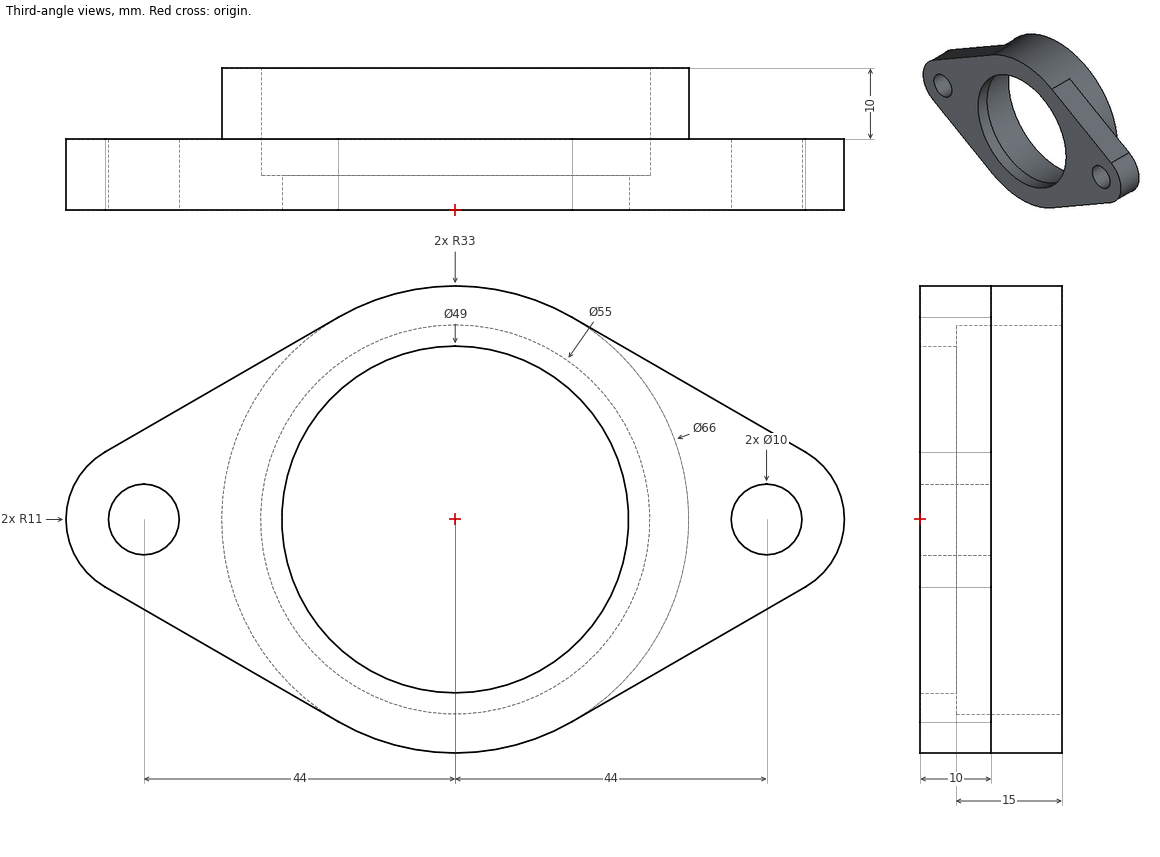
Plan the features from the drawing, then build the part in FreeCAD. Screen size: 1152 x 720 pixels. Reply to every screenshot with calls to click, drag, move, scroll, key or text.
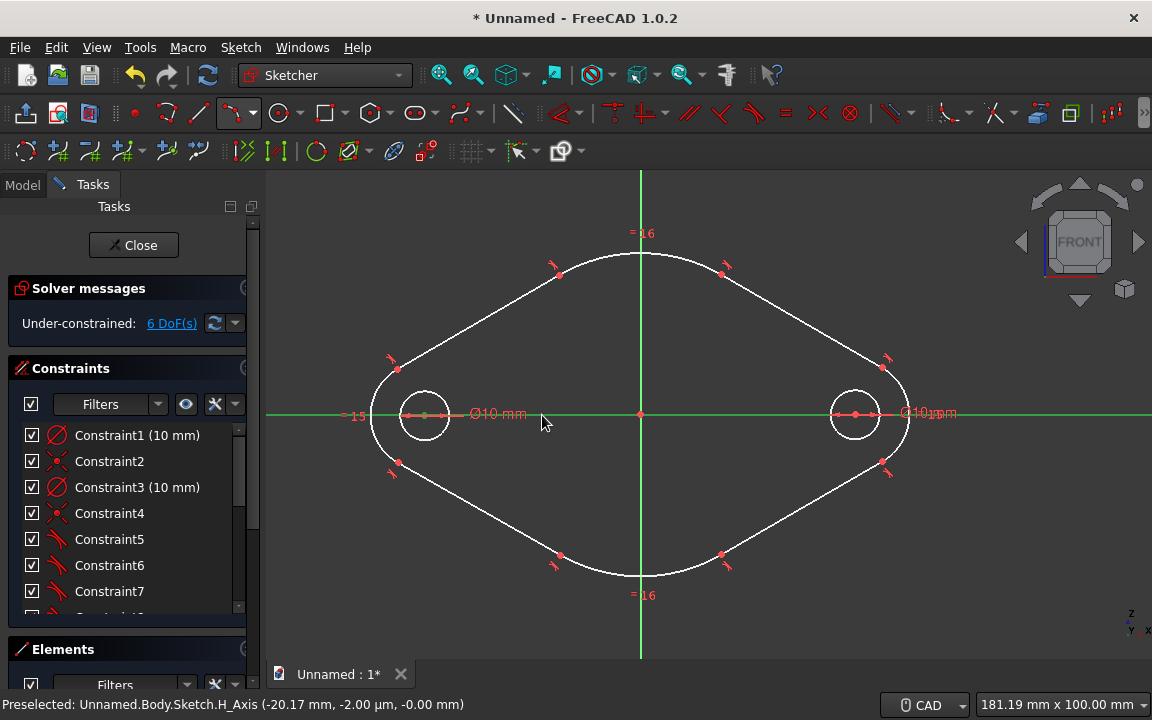
click(614, 114)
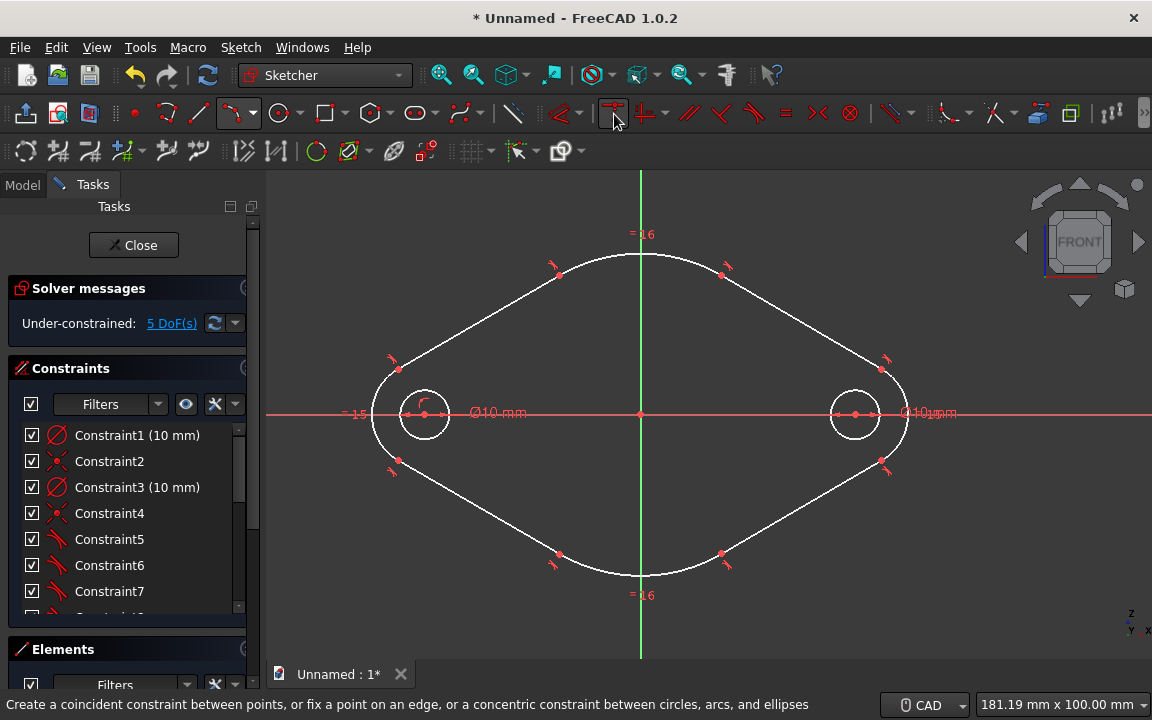
click(855, 415)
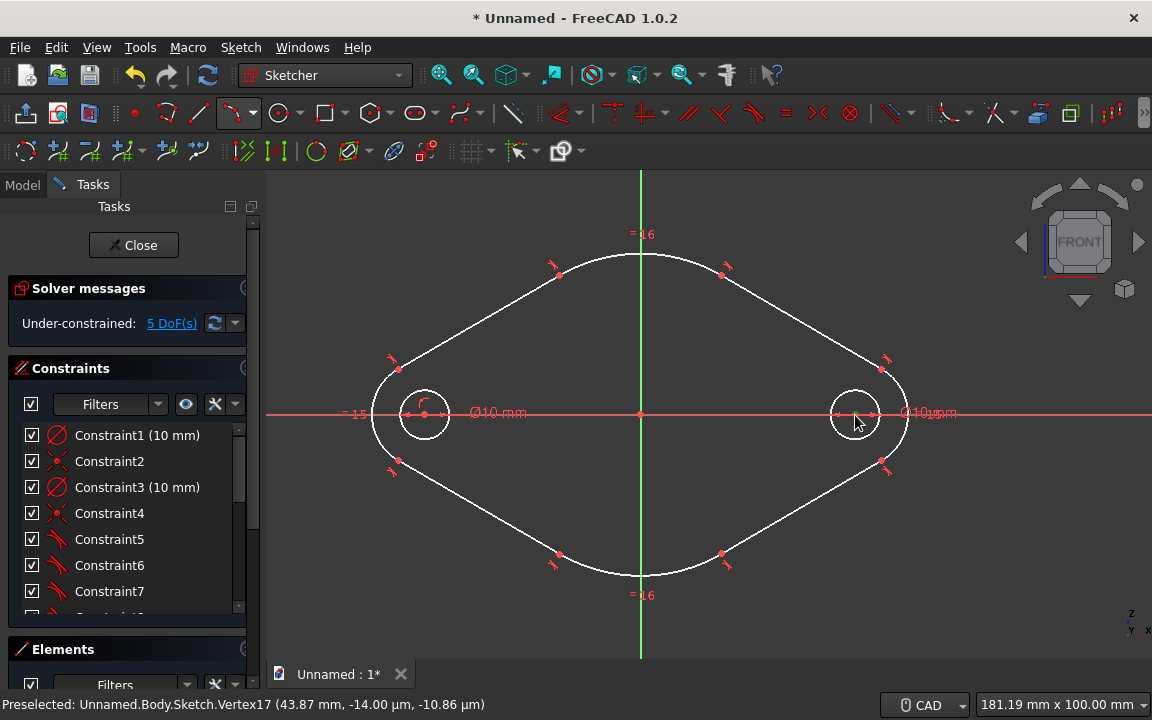
click(542, 415)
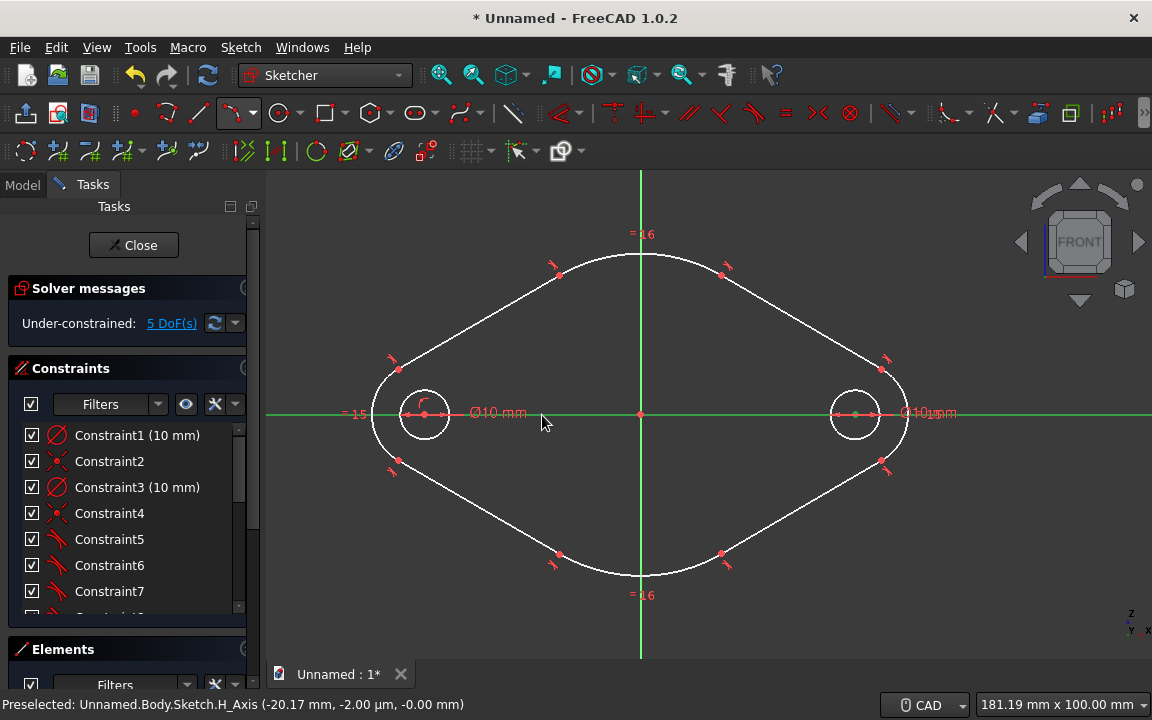
click(614, 114)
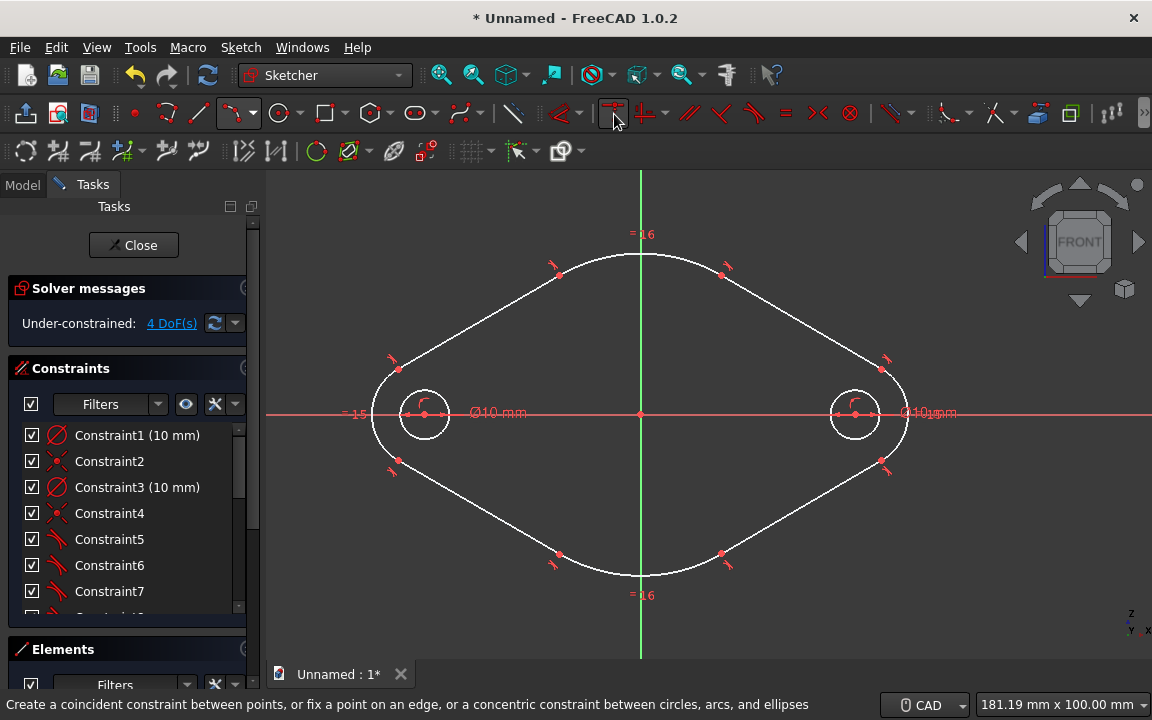
click(560, 114)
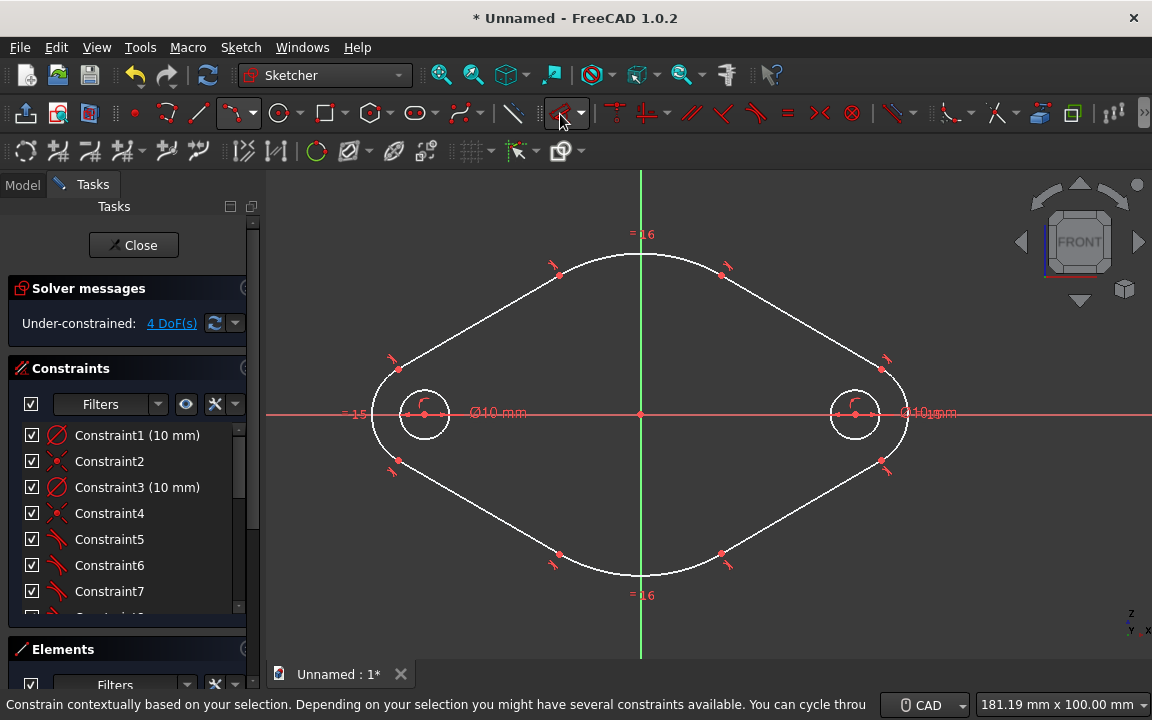
click(376, 393)
click(347, 380)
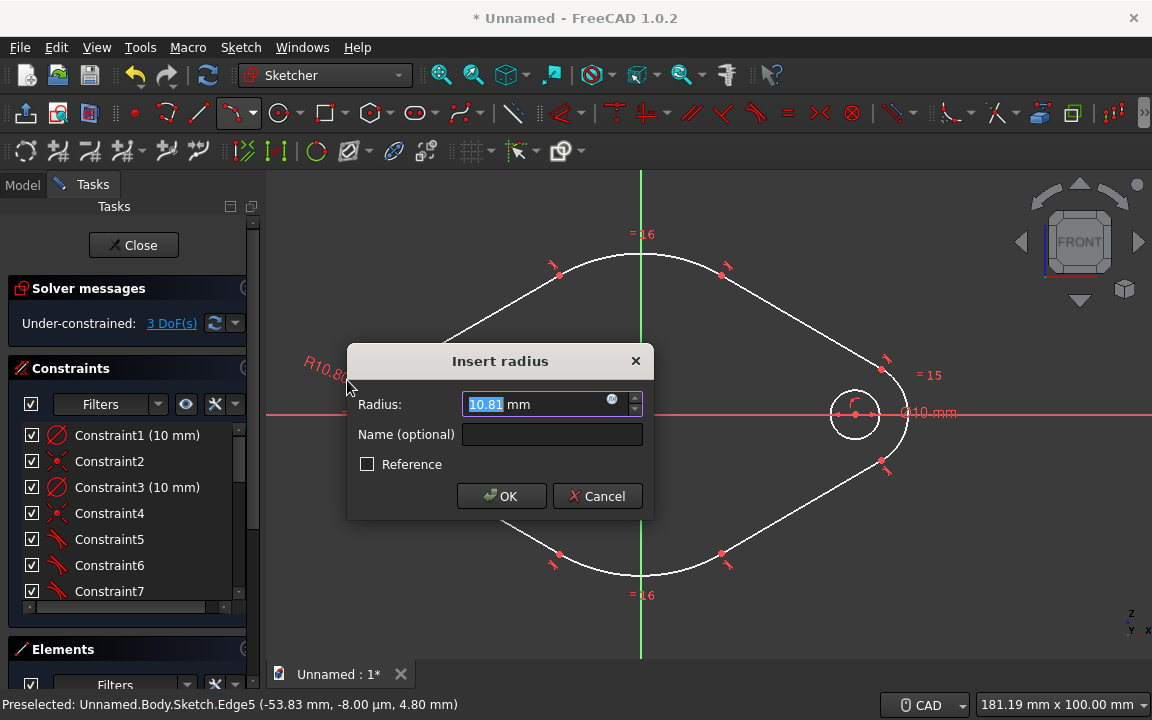
text(11)
key(Return)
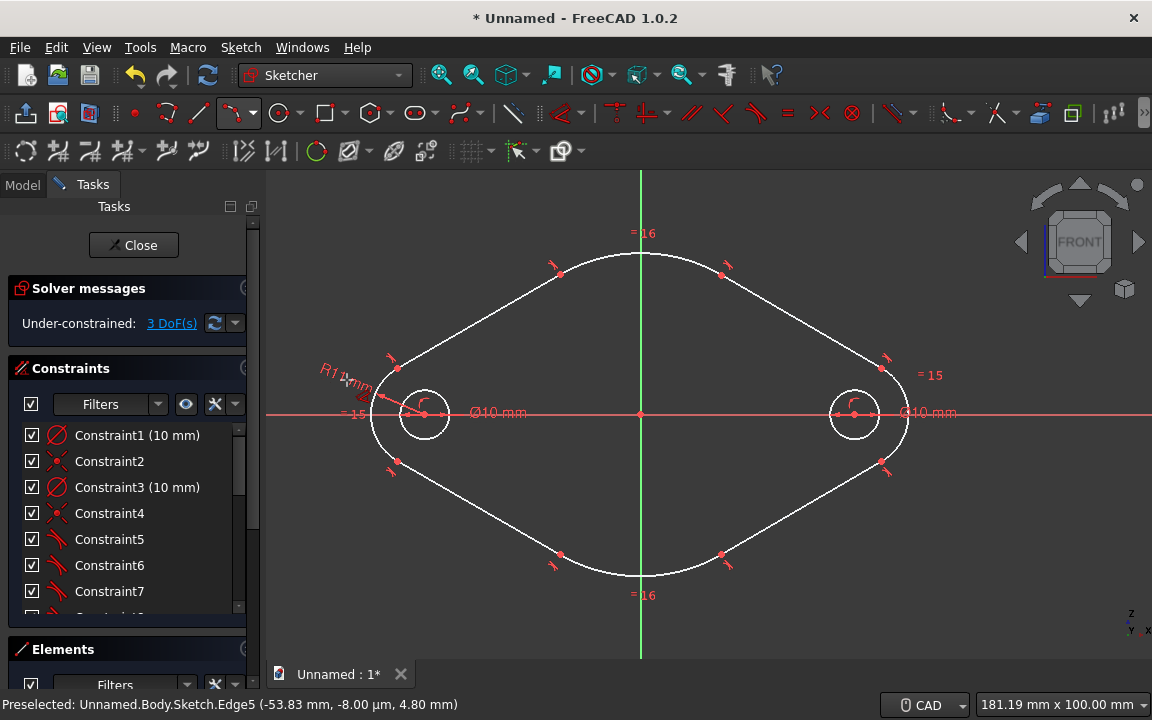
click(675, 257)
click(682, 226)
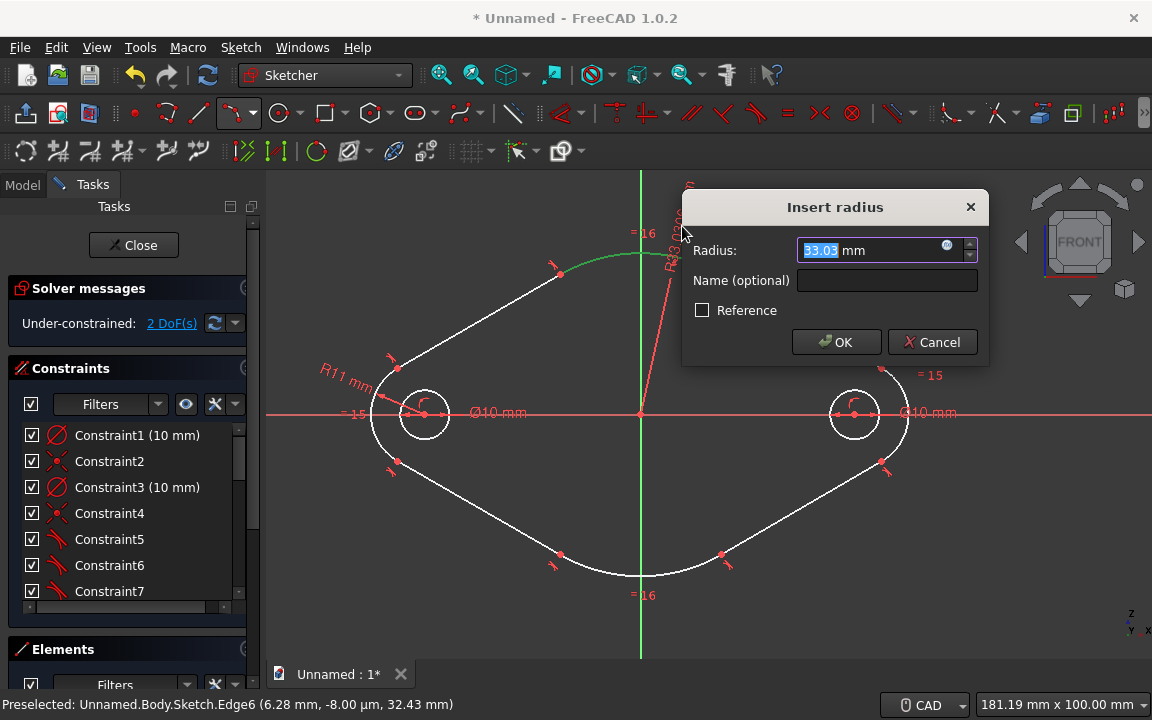
text(33)
key(Return)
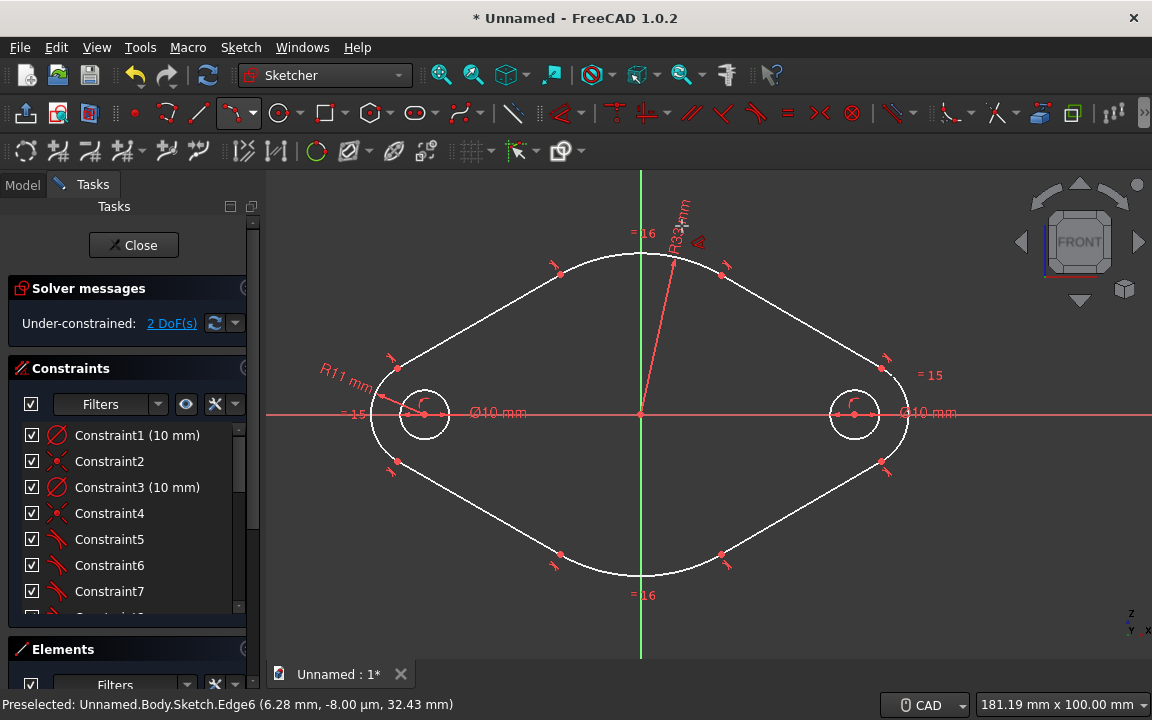
click(855, 415)
click(748, 449)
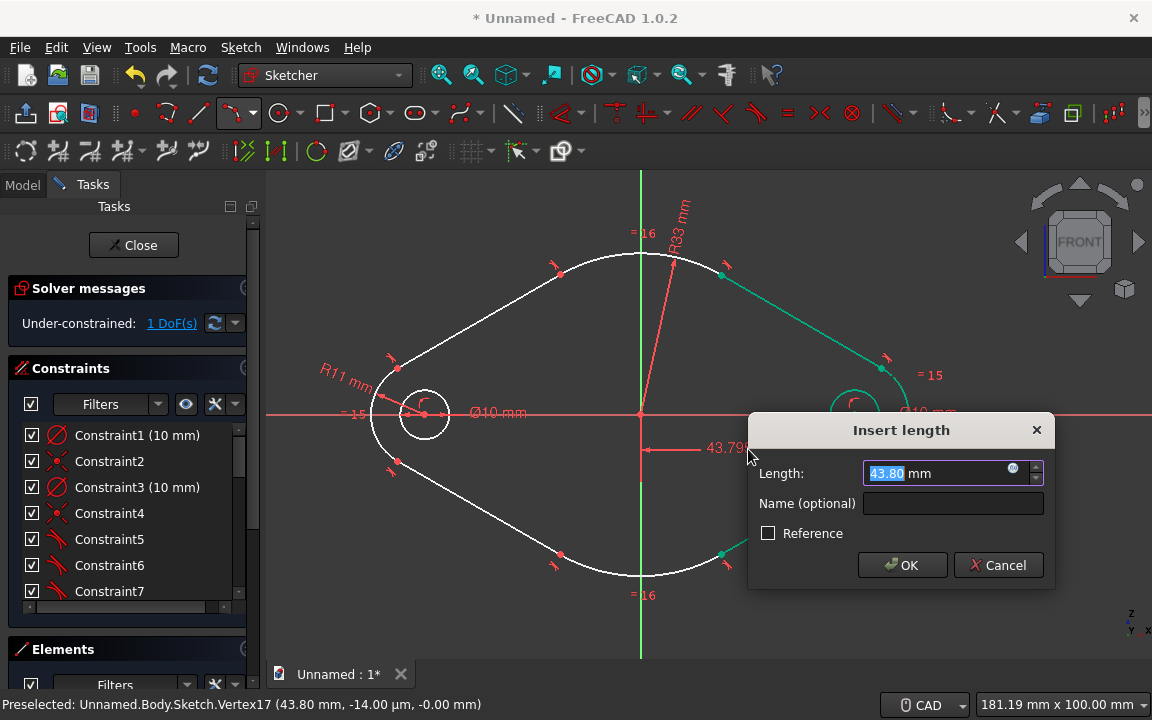
text(44)
key(Return)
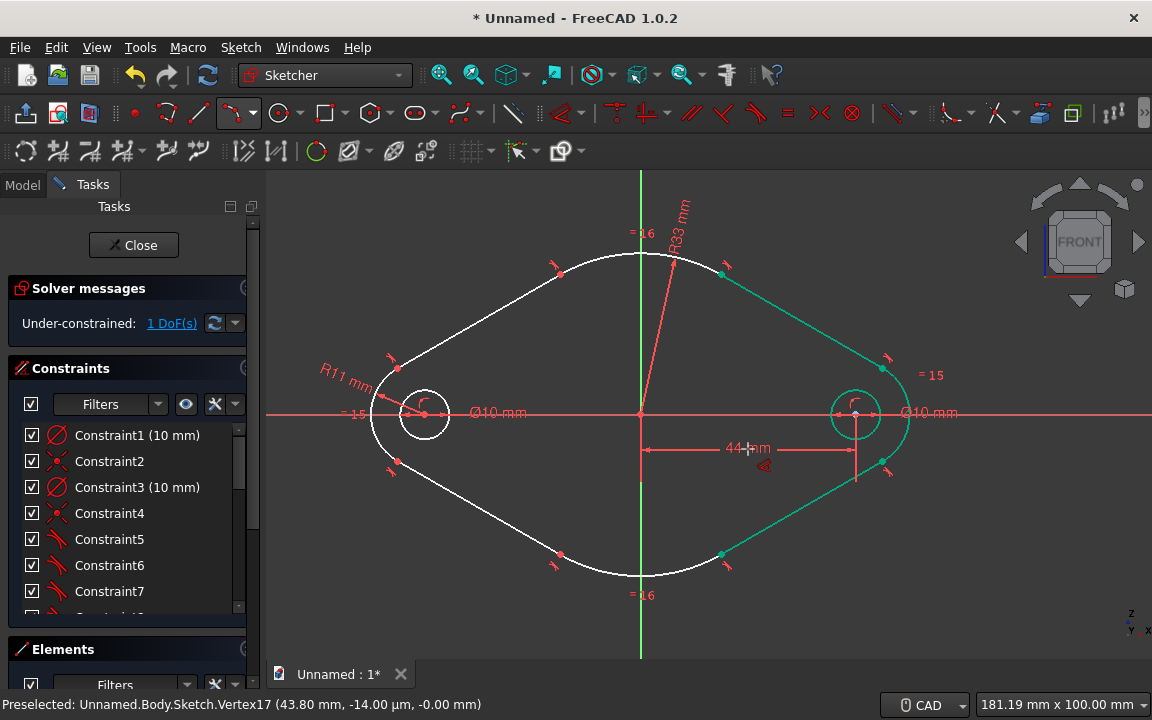
click(425, 415)
click(533, 449)